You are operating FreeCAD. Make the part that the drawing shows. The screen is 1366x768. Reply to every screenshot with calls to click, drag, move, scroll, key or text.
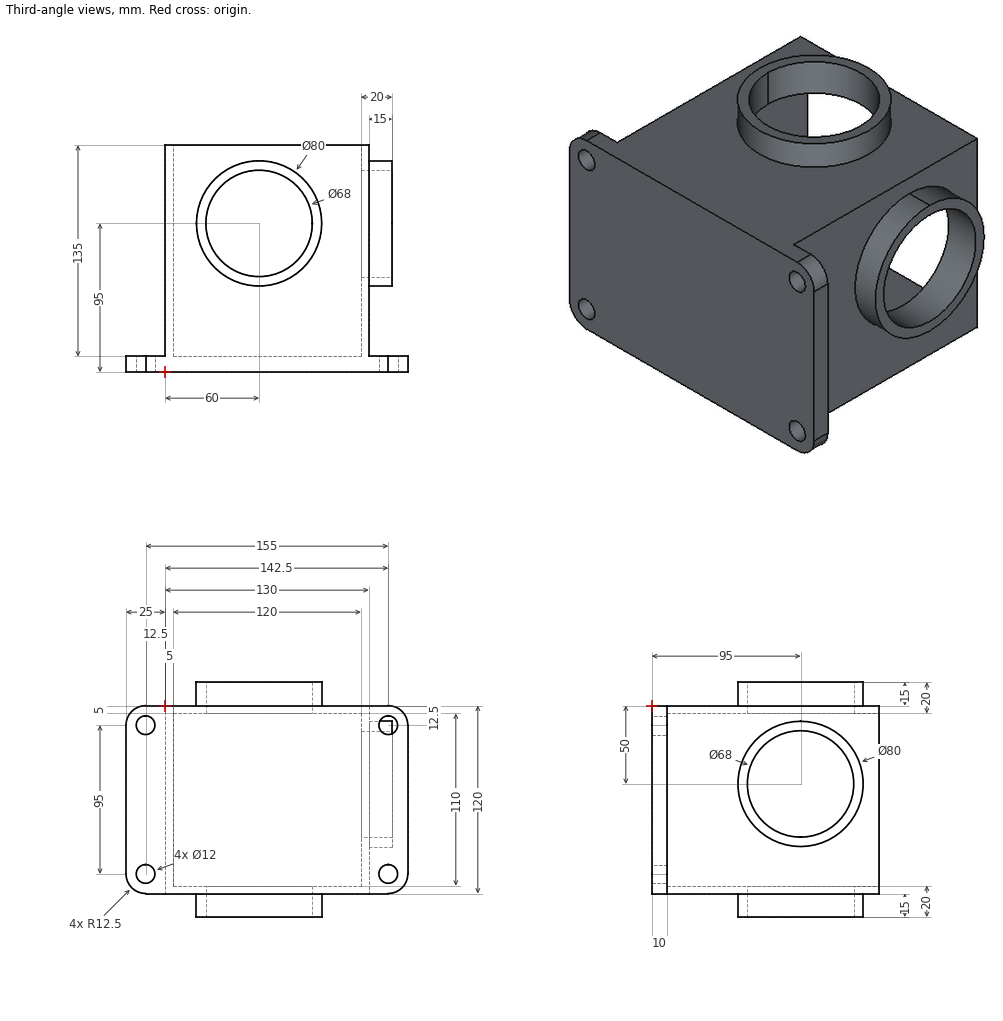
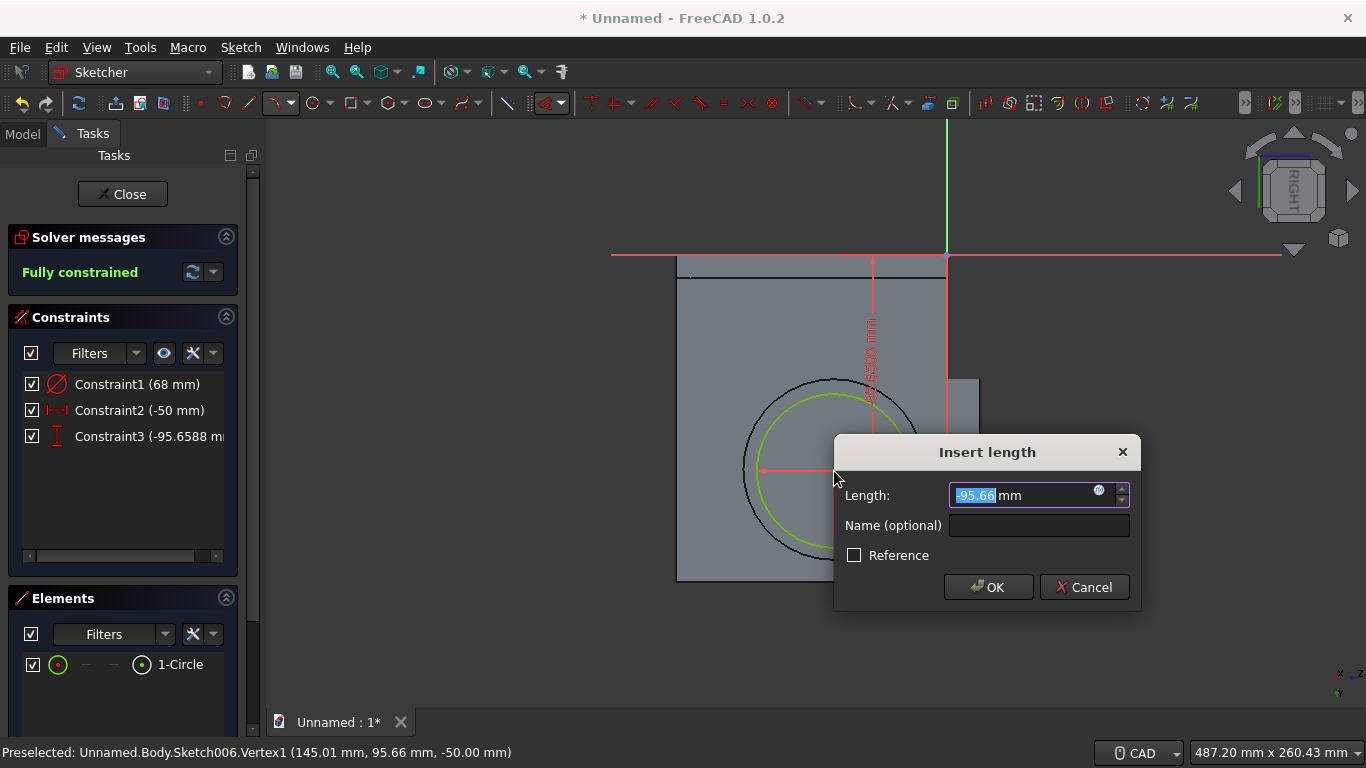
text(-95)
key(Return)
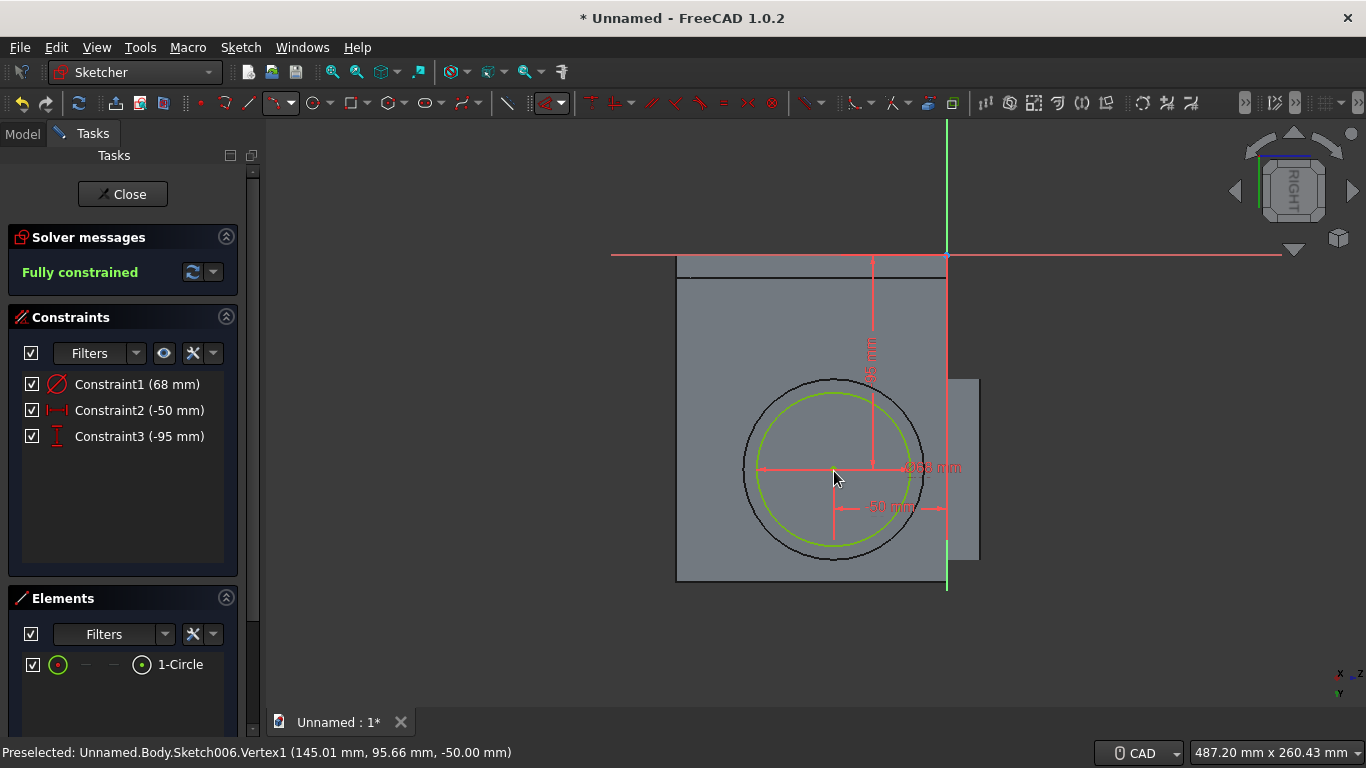
click(123, 194)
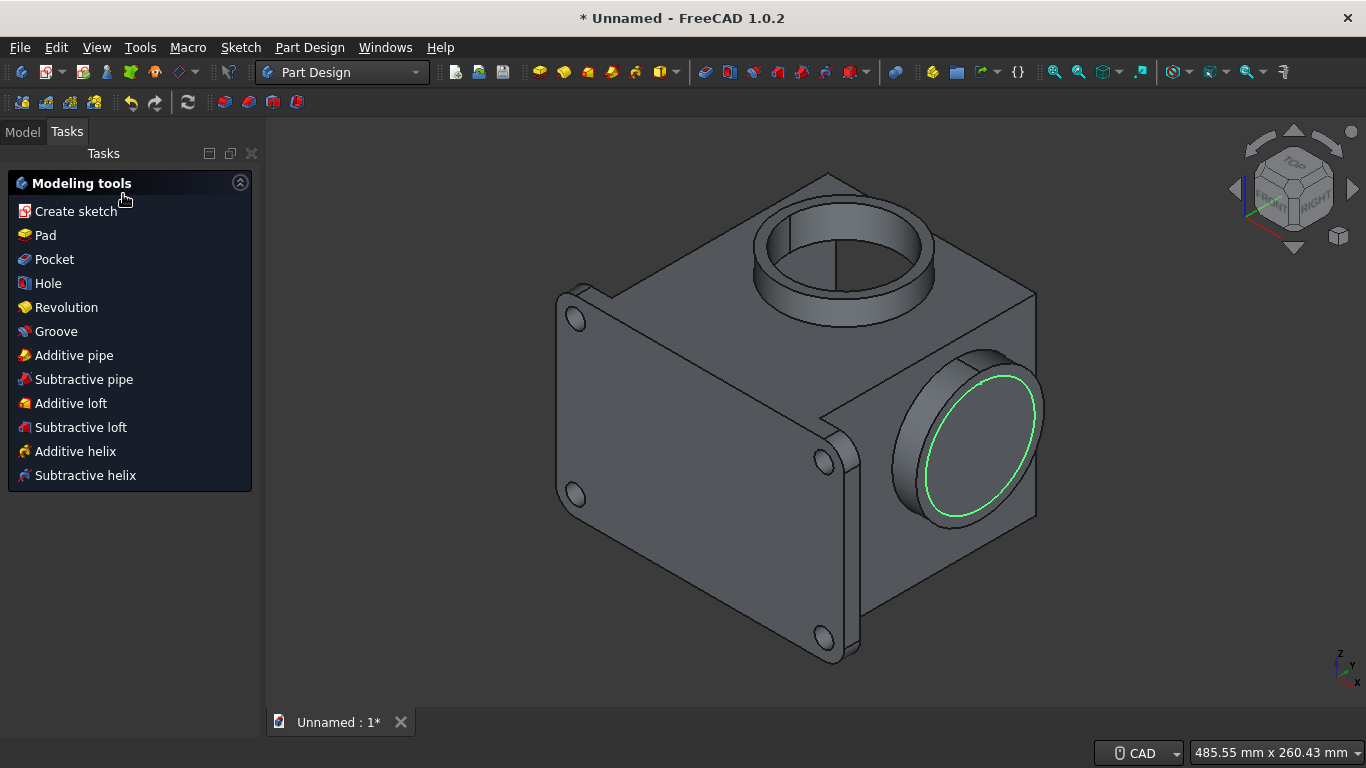
click(706, 72)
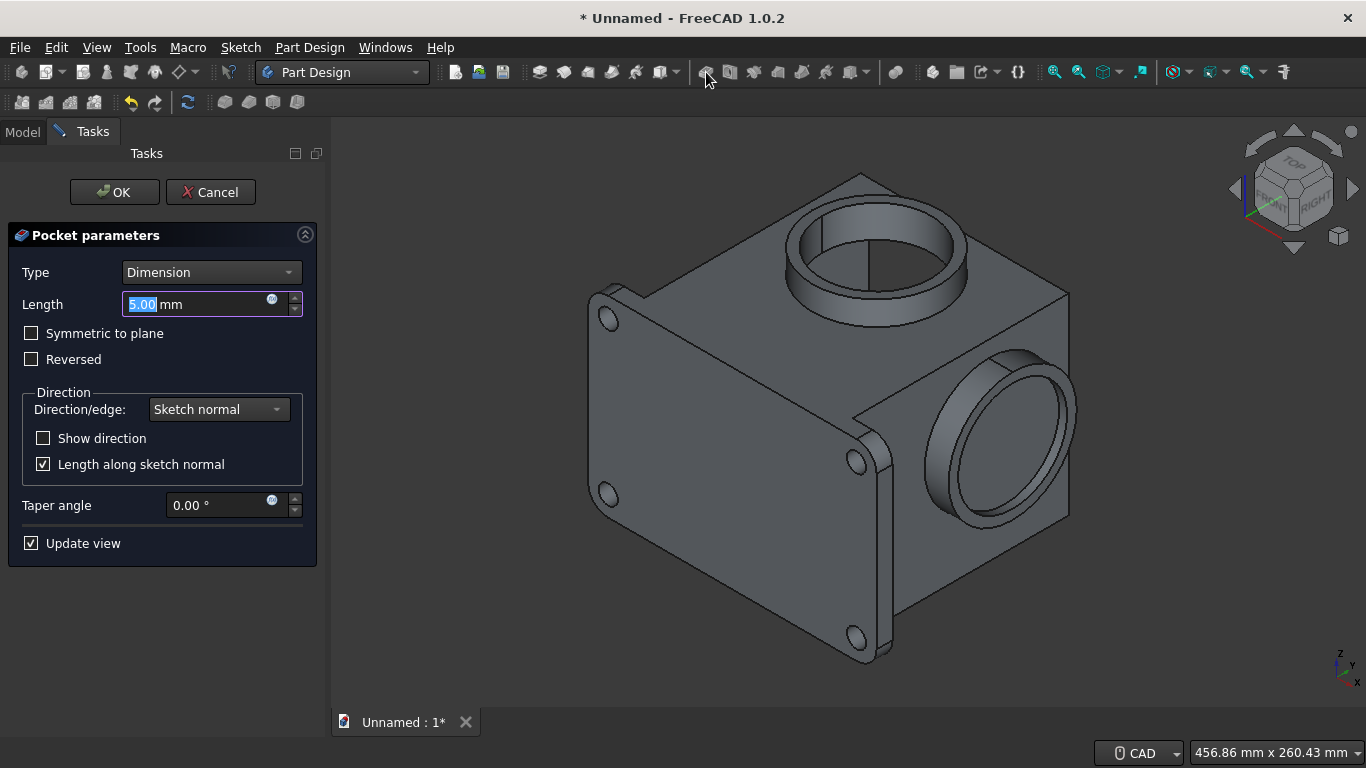
text(20)
key(Tab)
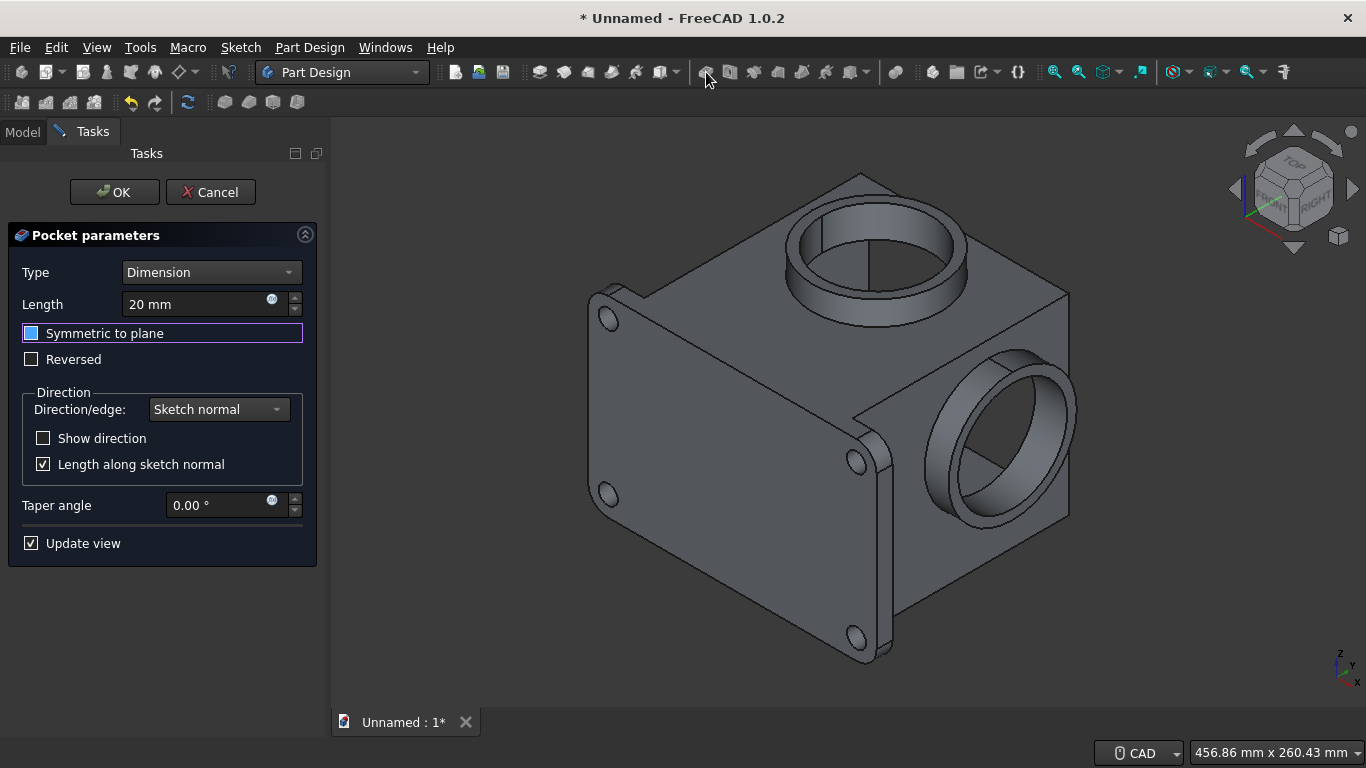
click(115, 192)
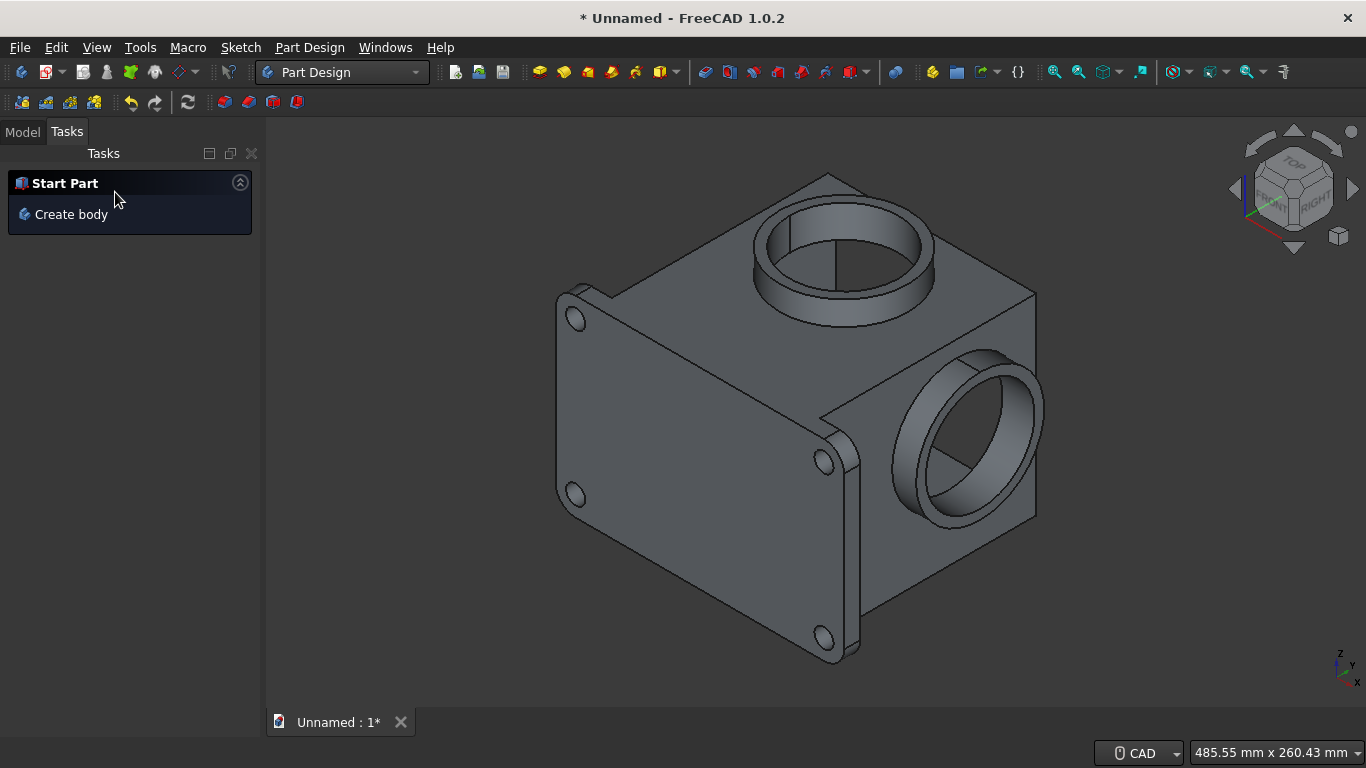
click(23, 131)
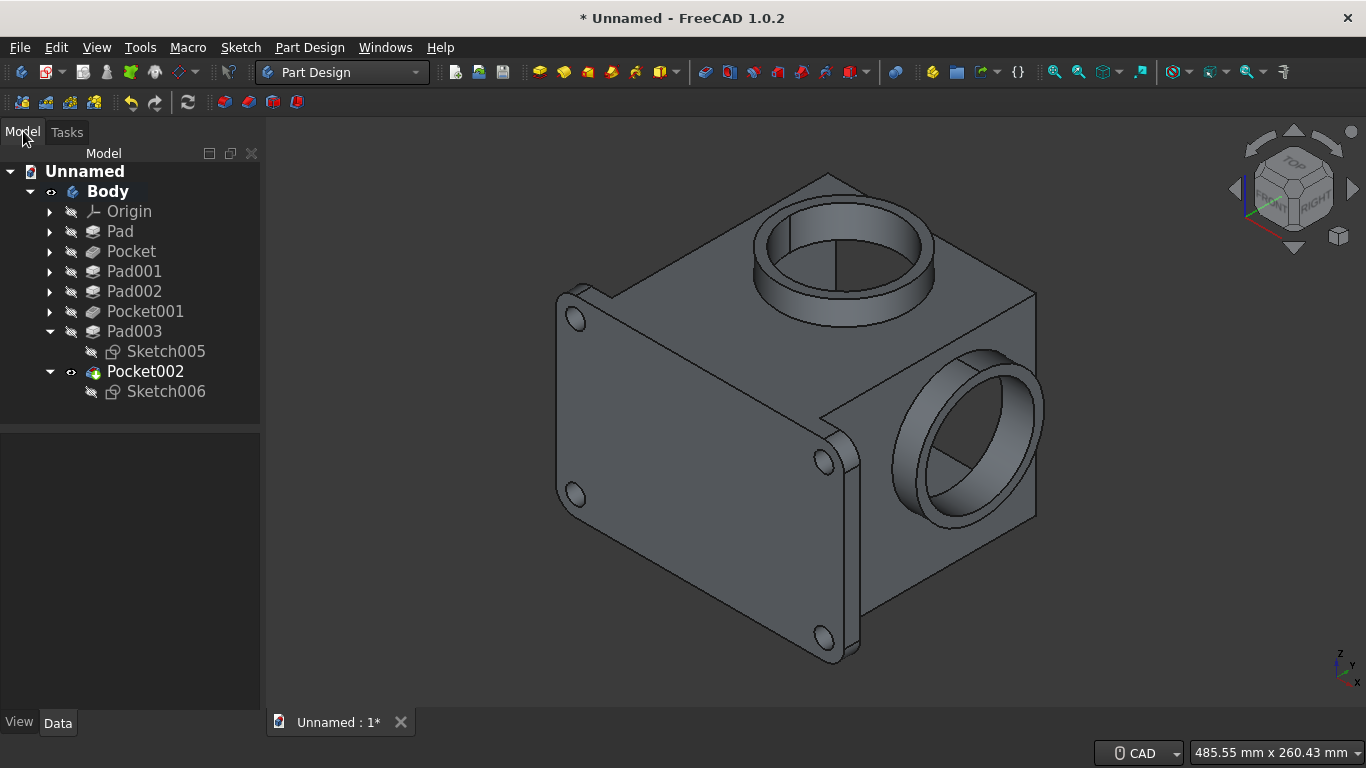
click(50, 212)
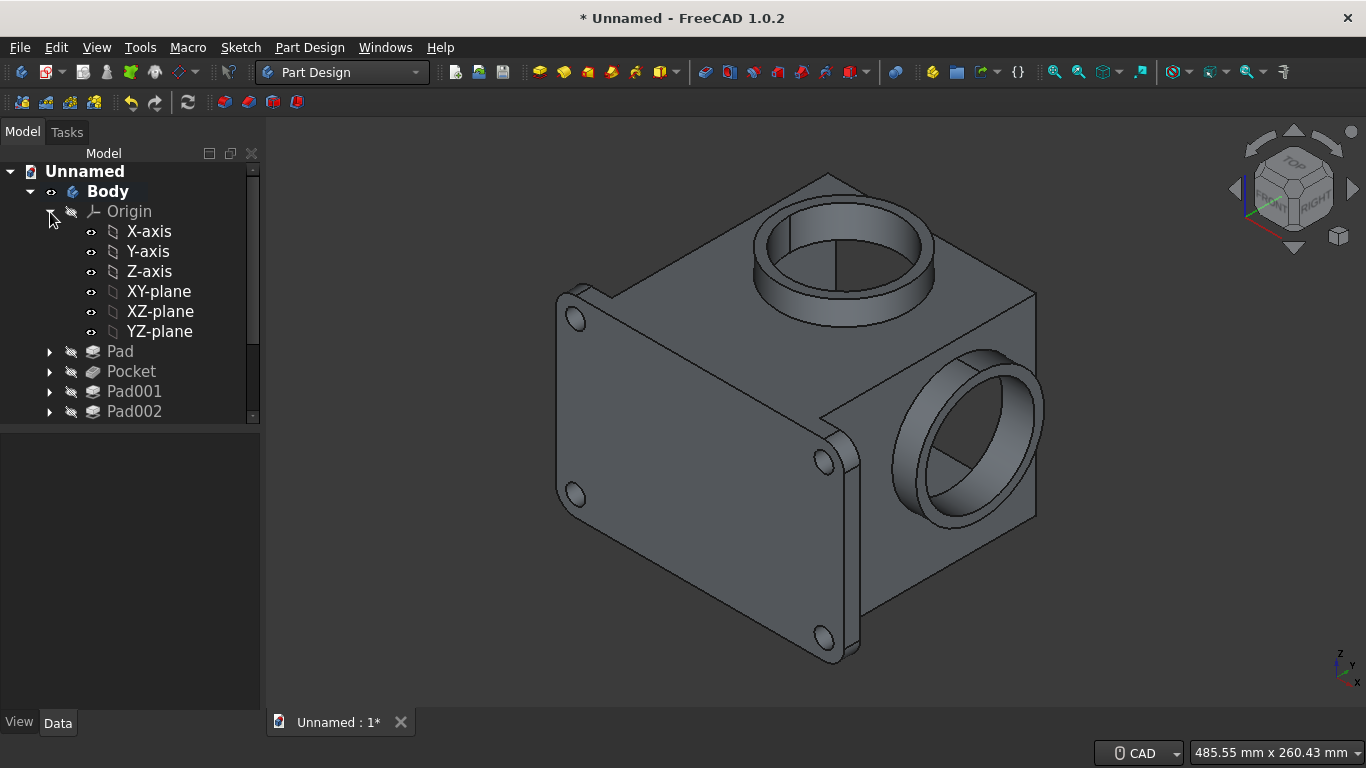
click(136, 292)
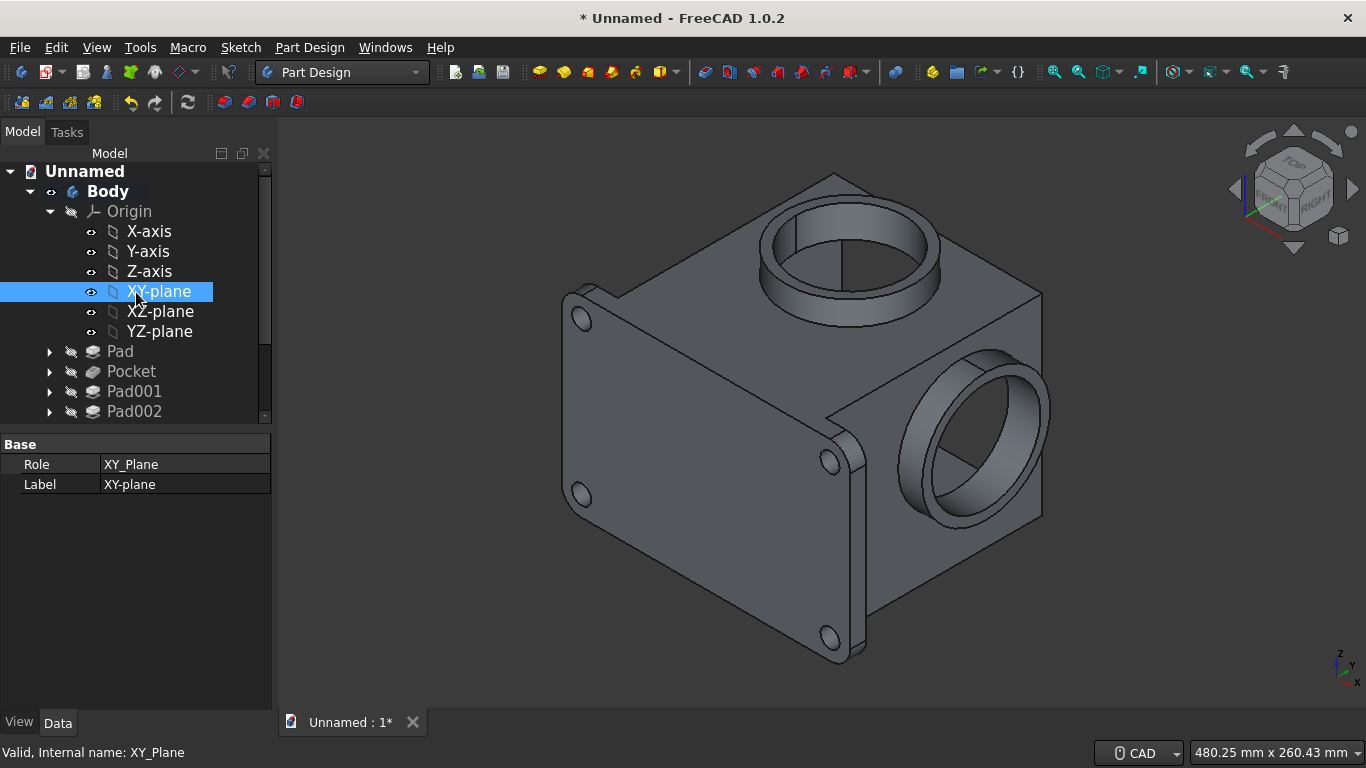
click(180, 72)